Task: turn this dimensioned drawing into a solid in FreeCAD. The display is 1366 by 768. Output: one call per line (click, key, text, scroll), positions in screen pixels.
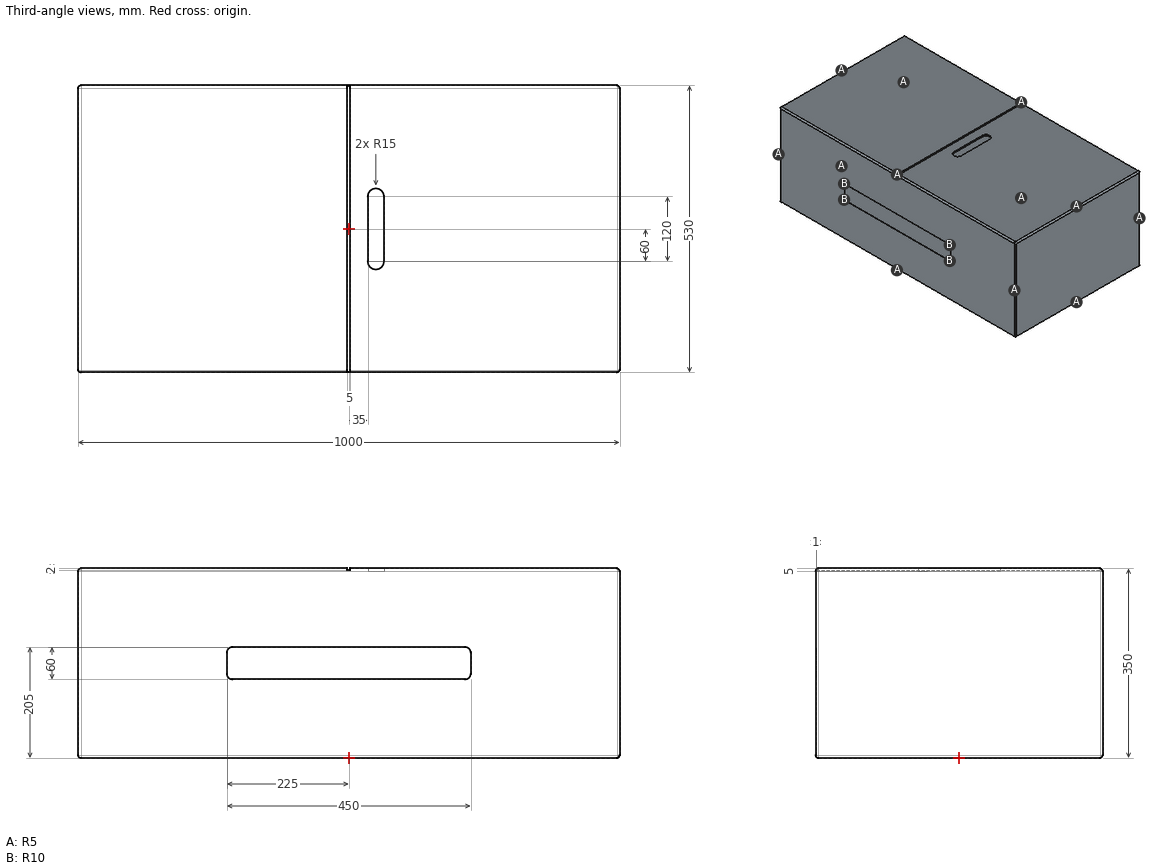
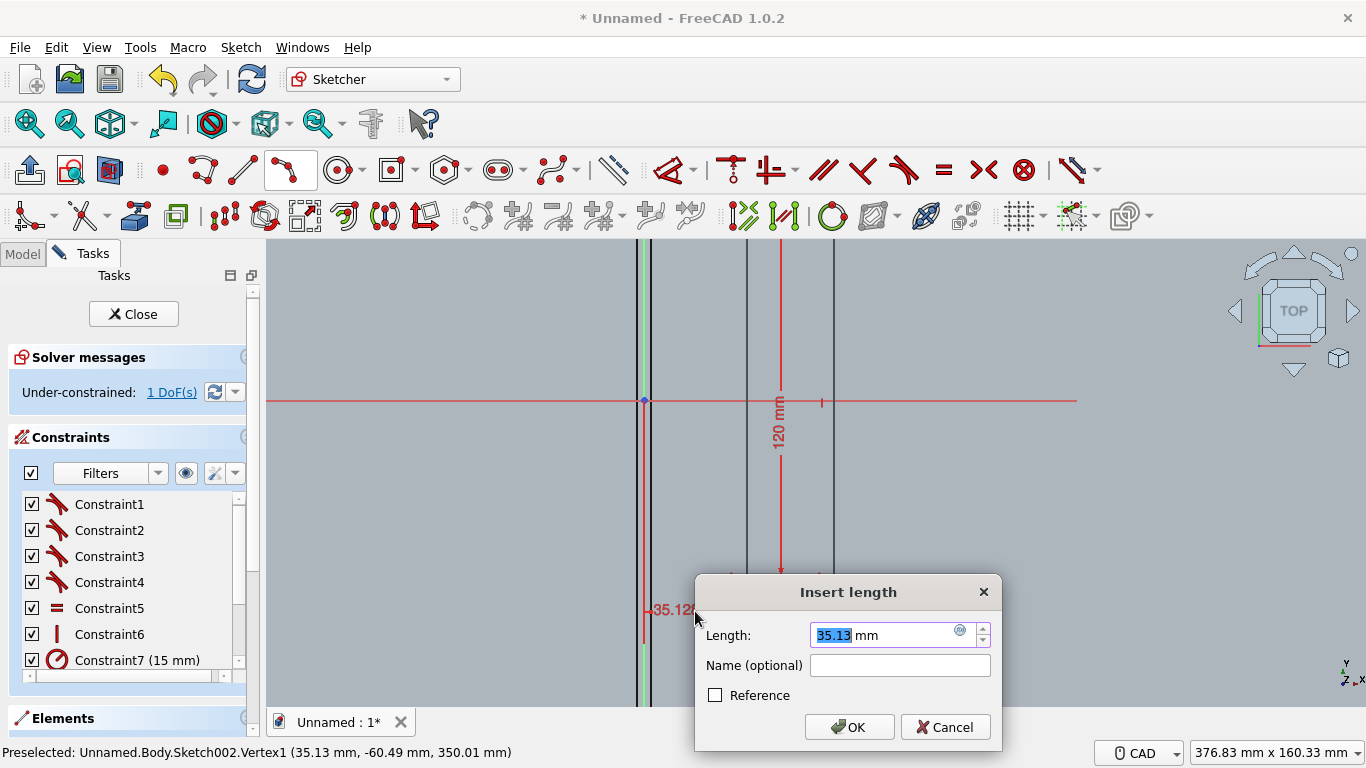
text(35)
key(Return)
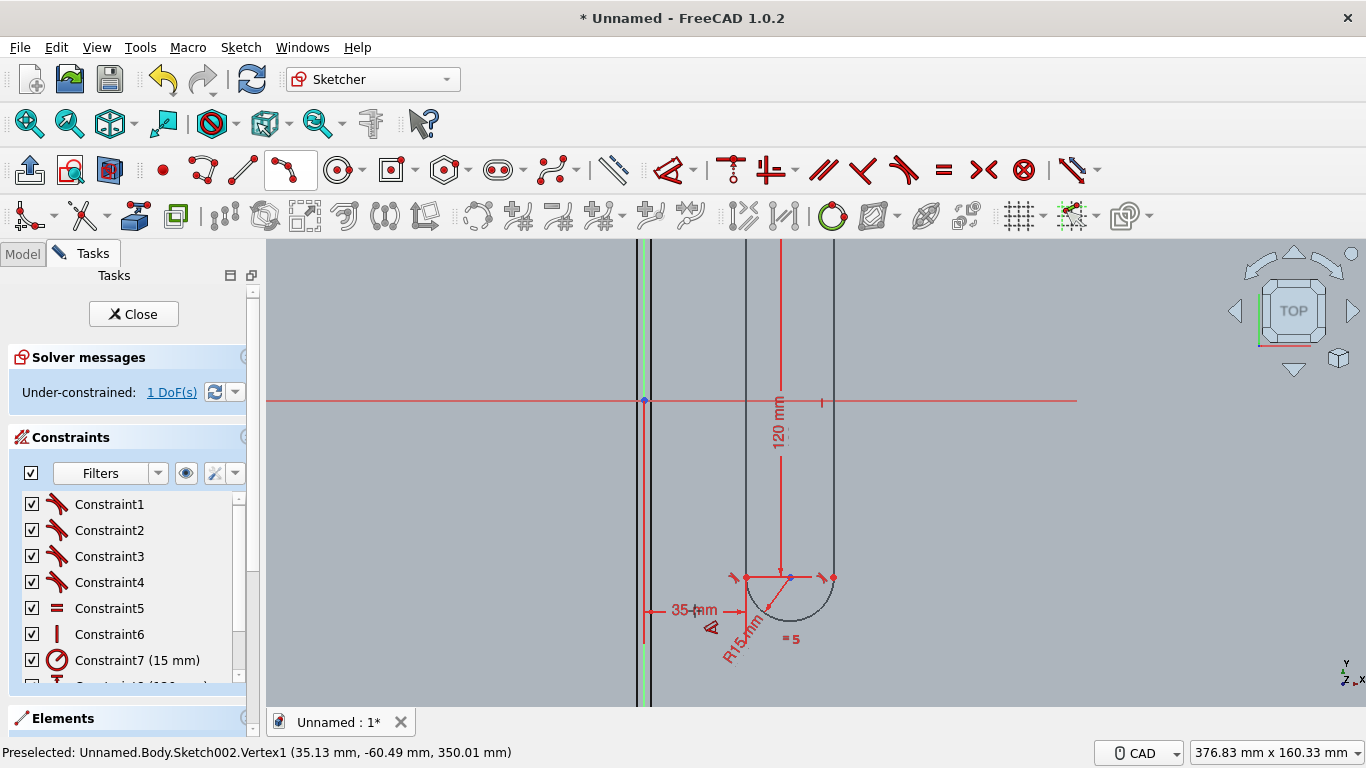
click(746, 577)
click(610, 489)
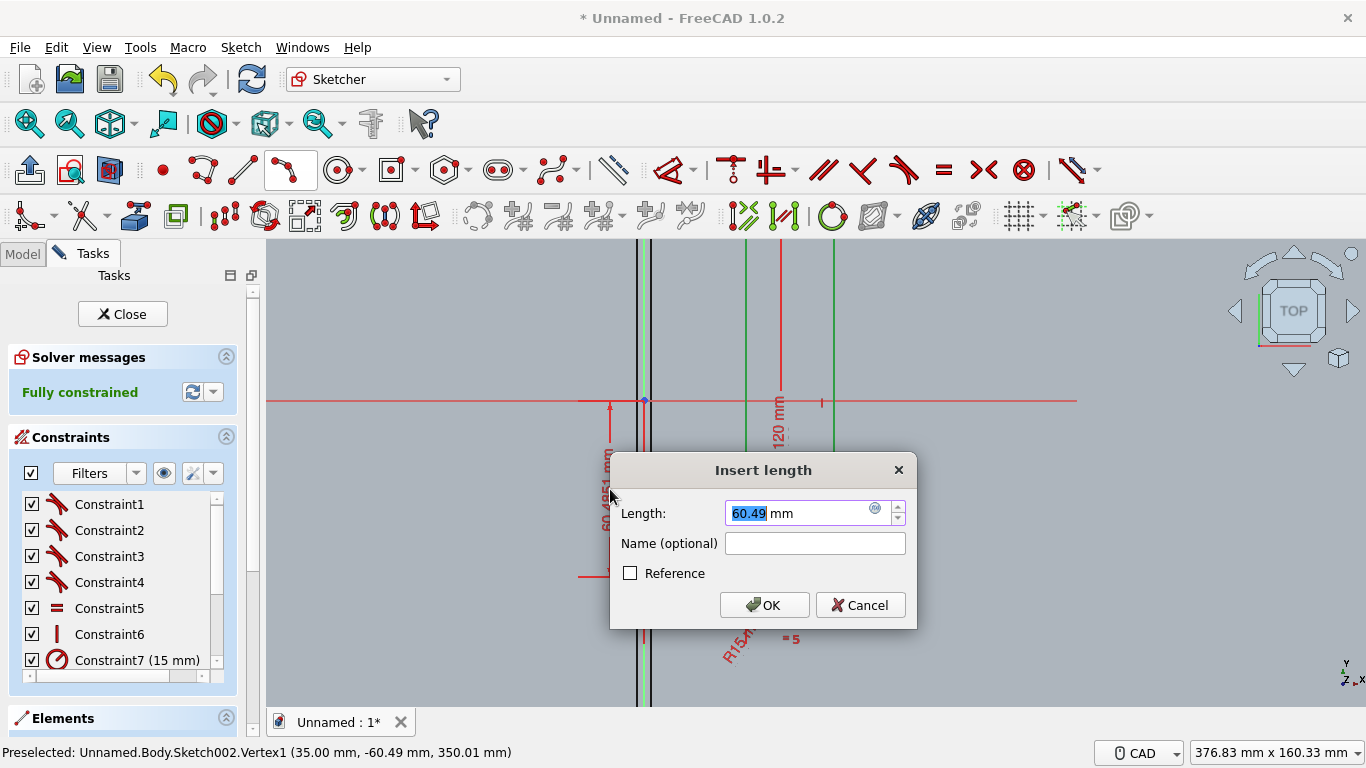
text(60)
key(Return)
key(Escape)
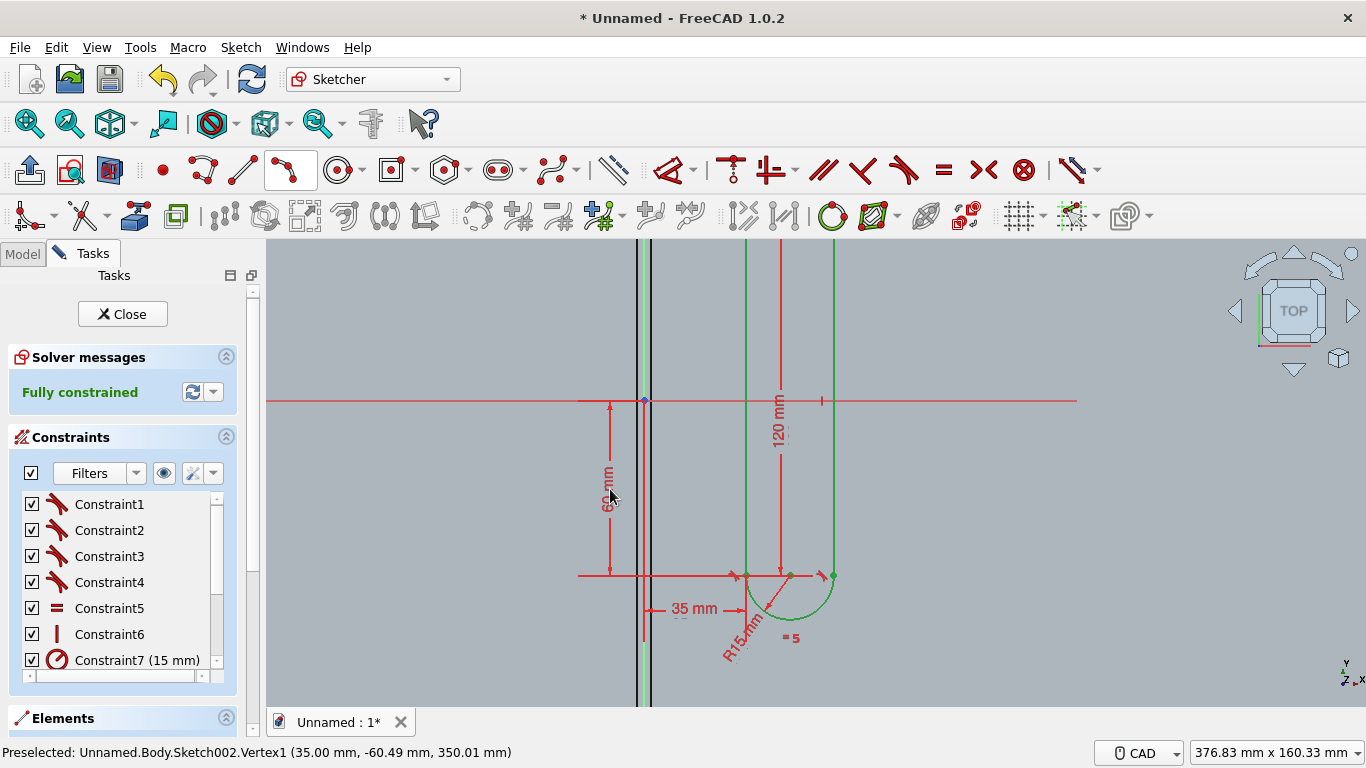
click(123, 314)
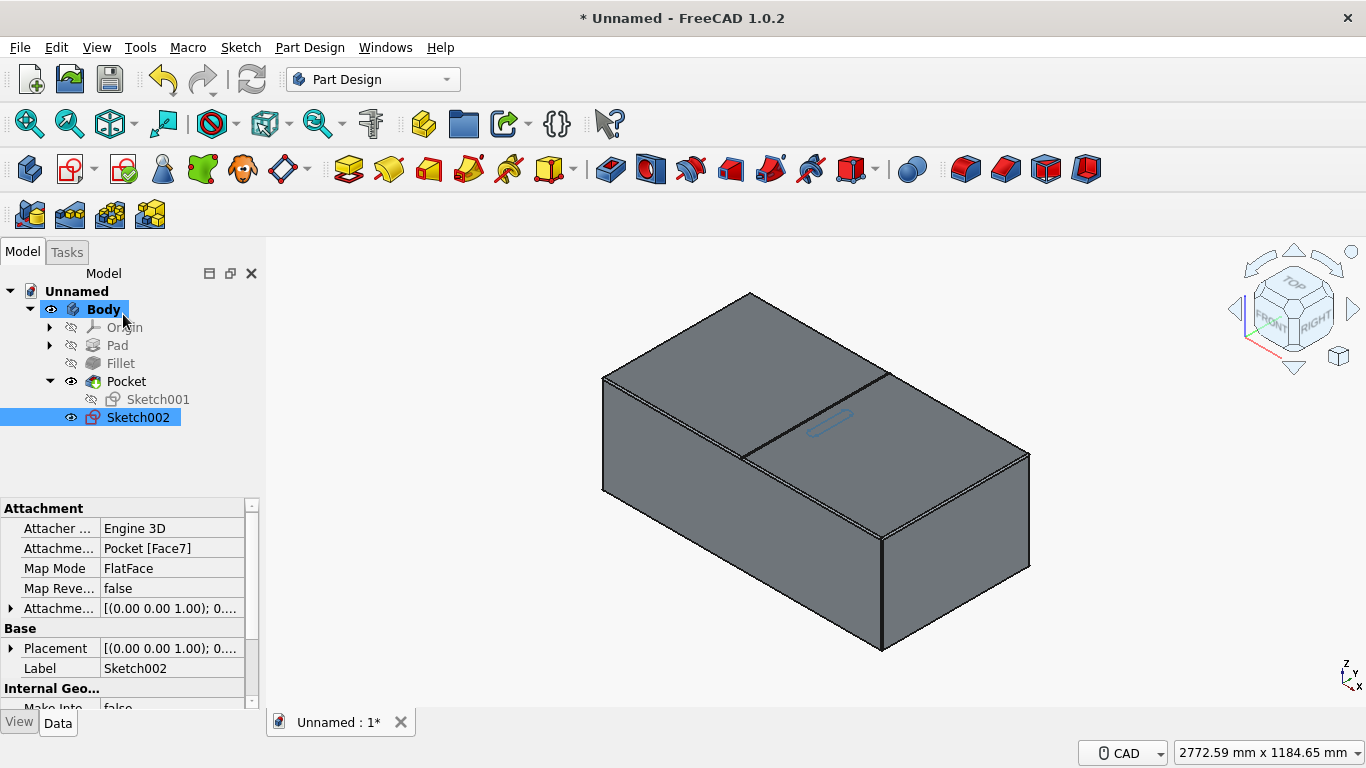
click(612, 170)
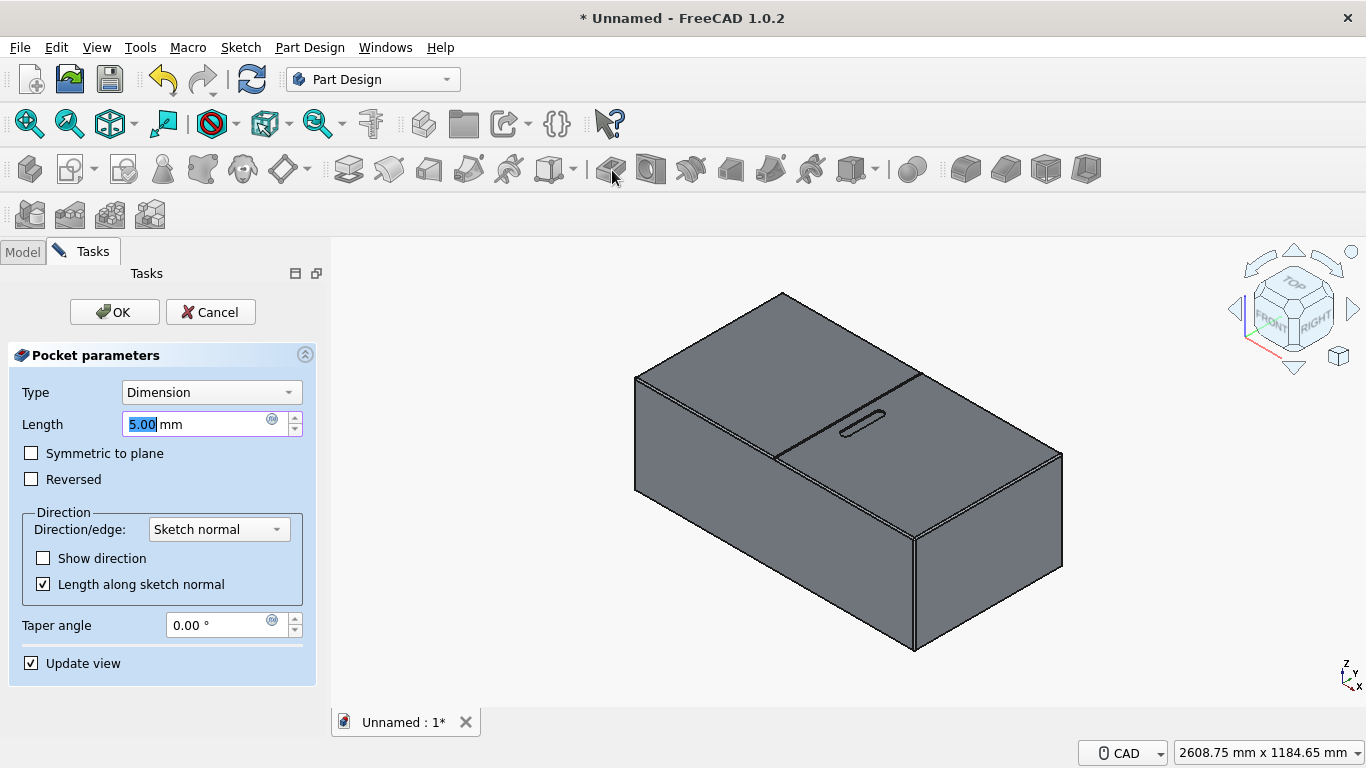
text(5)
key(Tab)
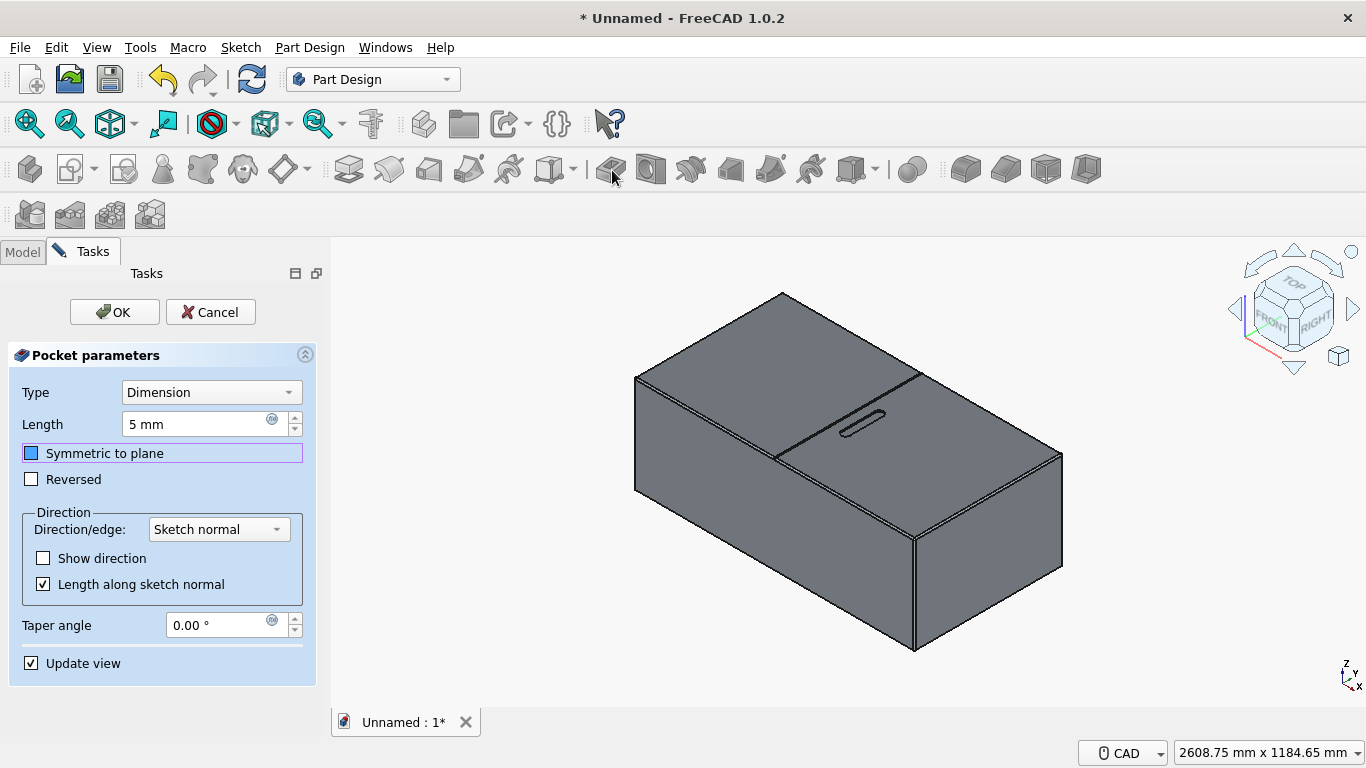
click(115, 312)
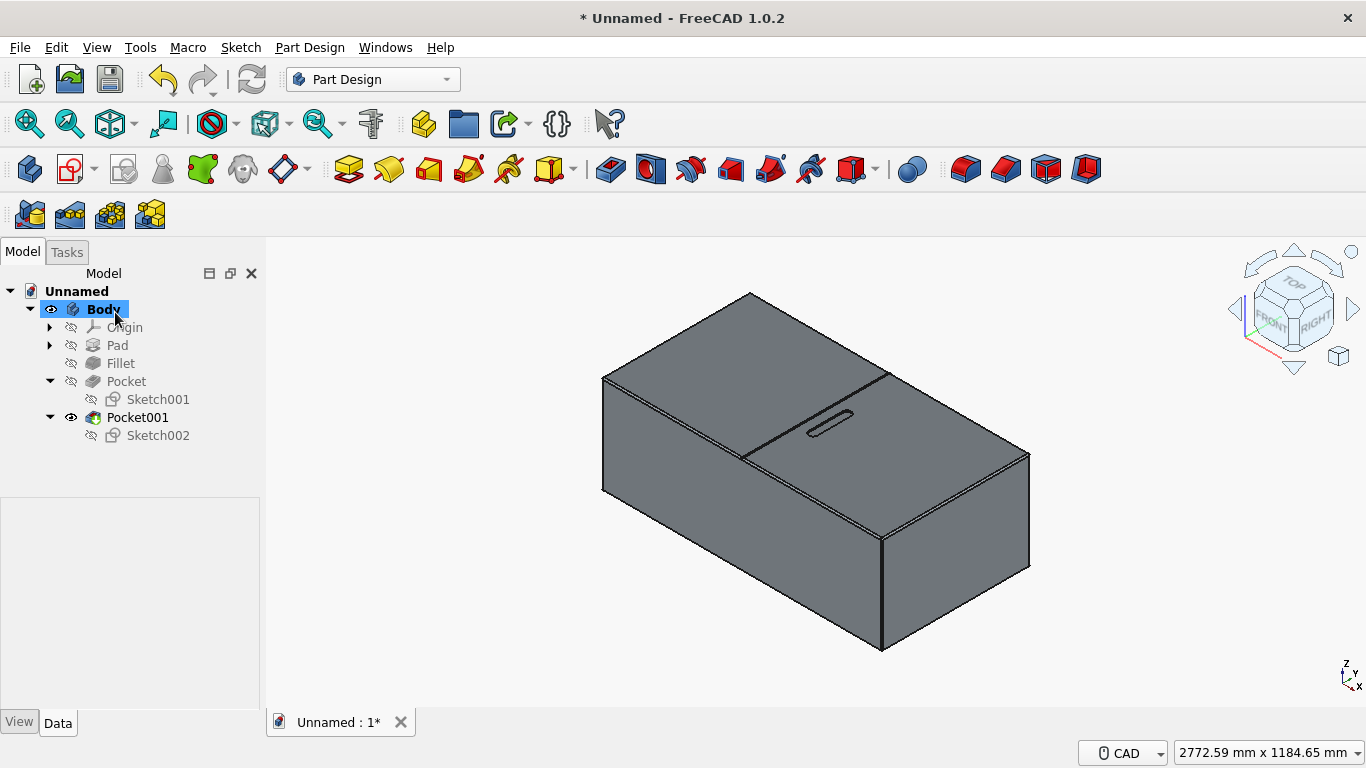
click(821, 560)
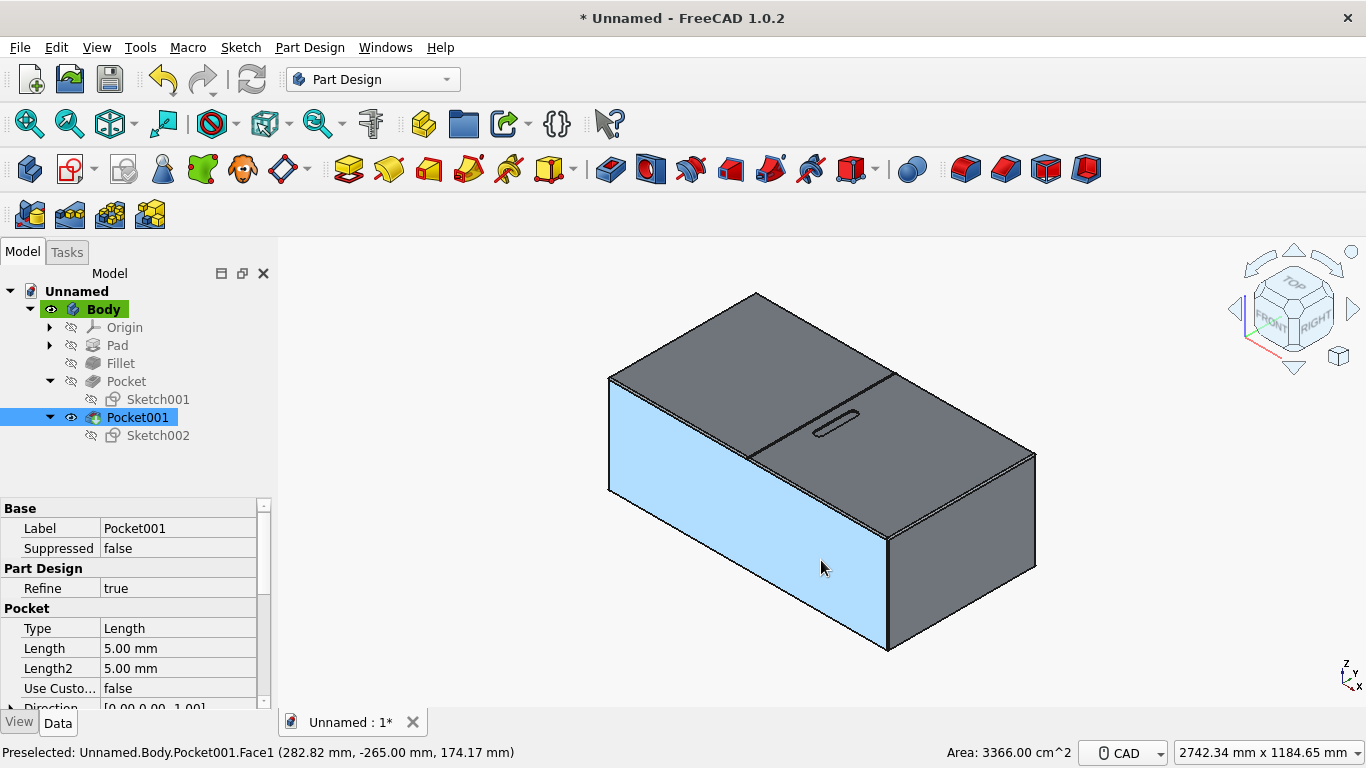
click(70, 170)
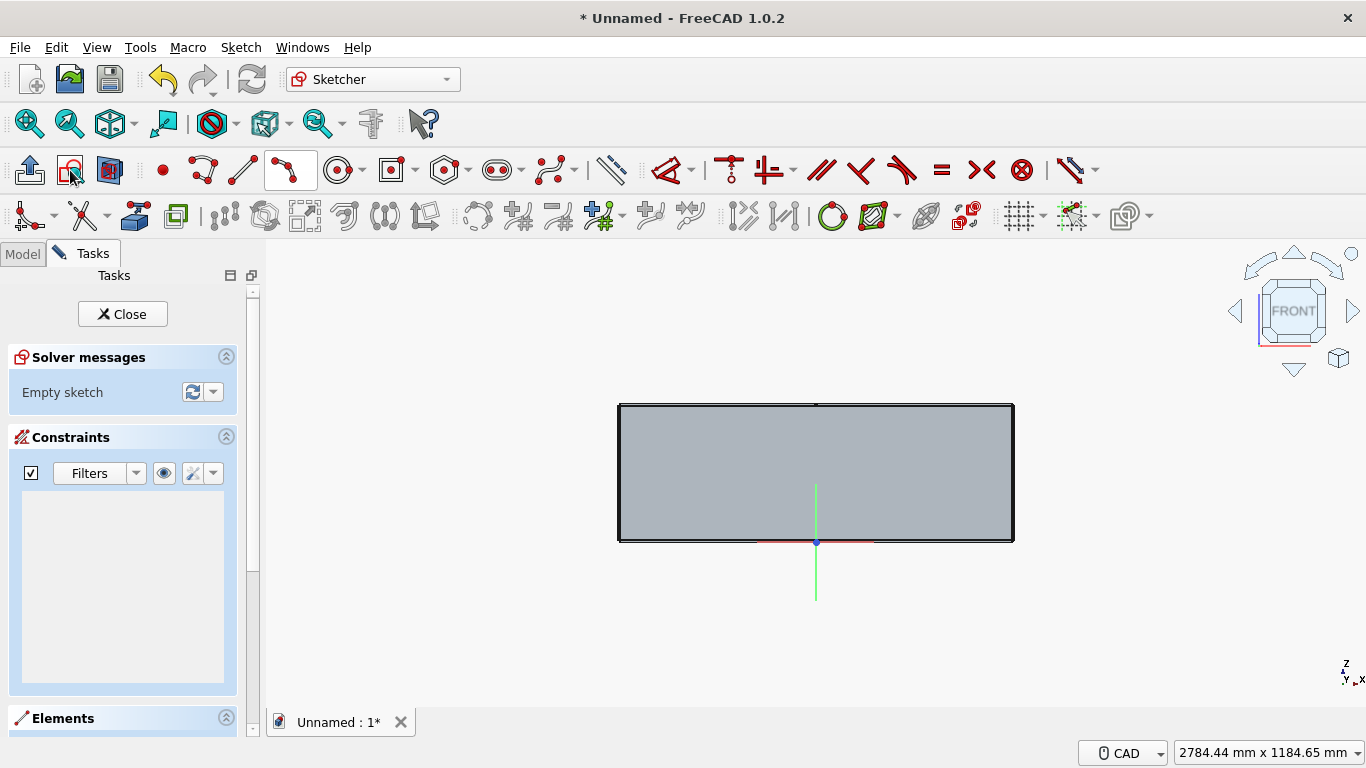
scroll(846, 514, up, 6)